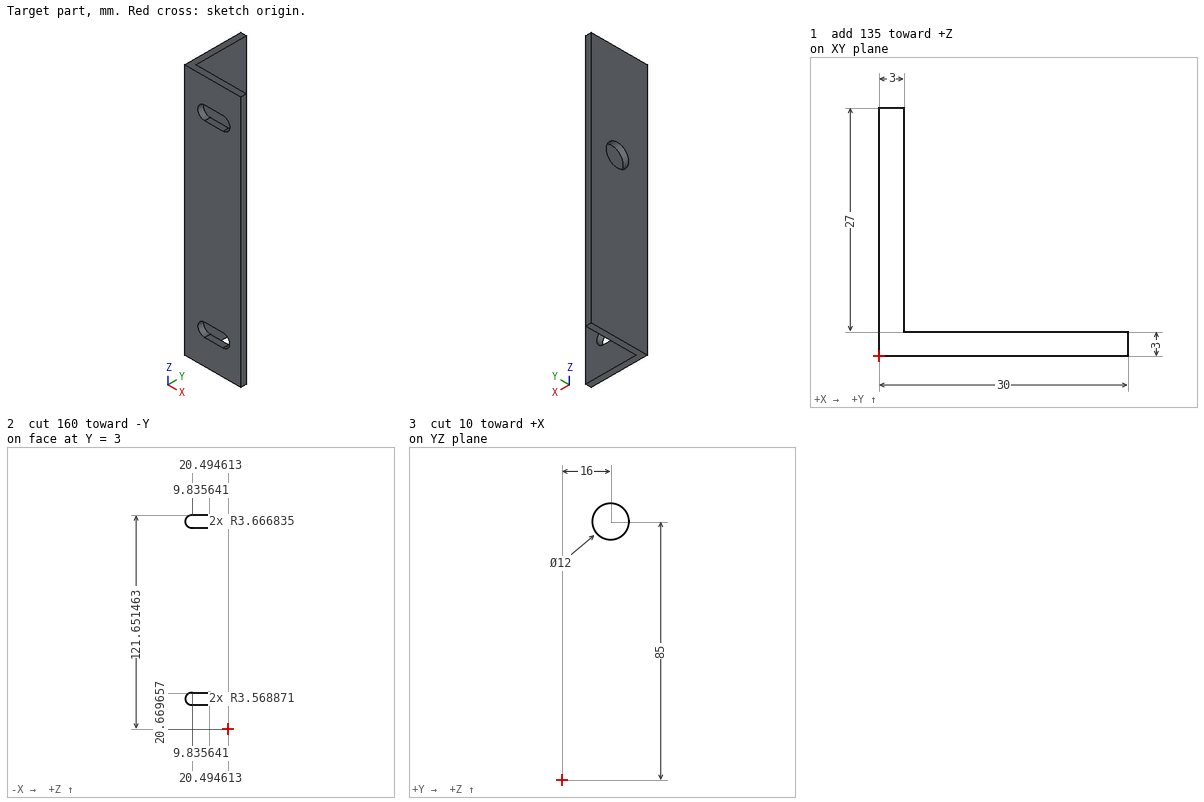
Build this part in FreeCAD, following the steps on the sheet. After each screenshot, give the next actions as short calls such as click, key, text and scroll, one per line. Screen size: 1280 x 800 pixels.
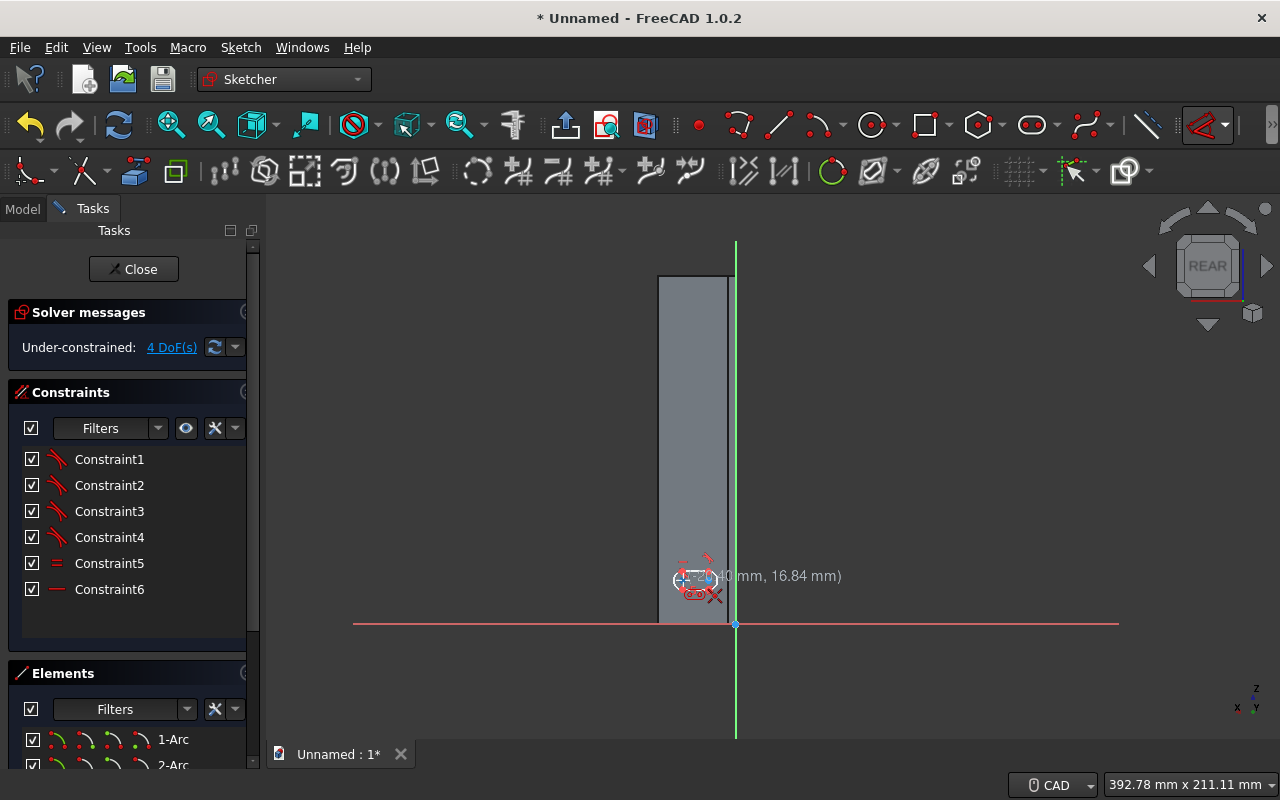
scroll(683, 320, up, 5)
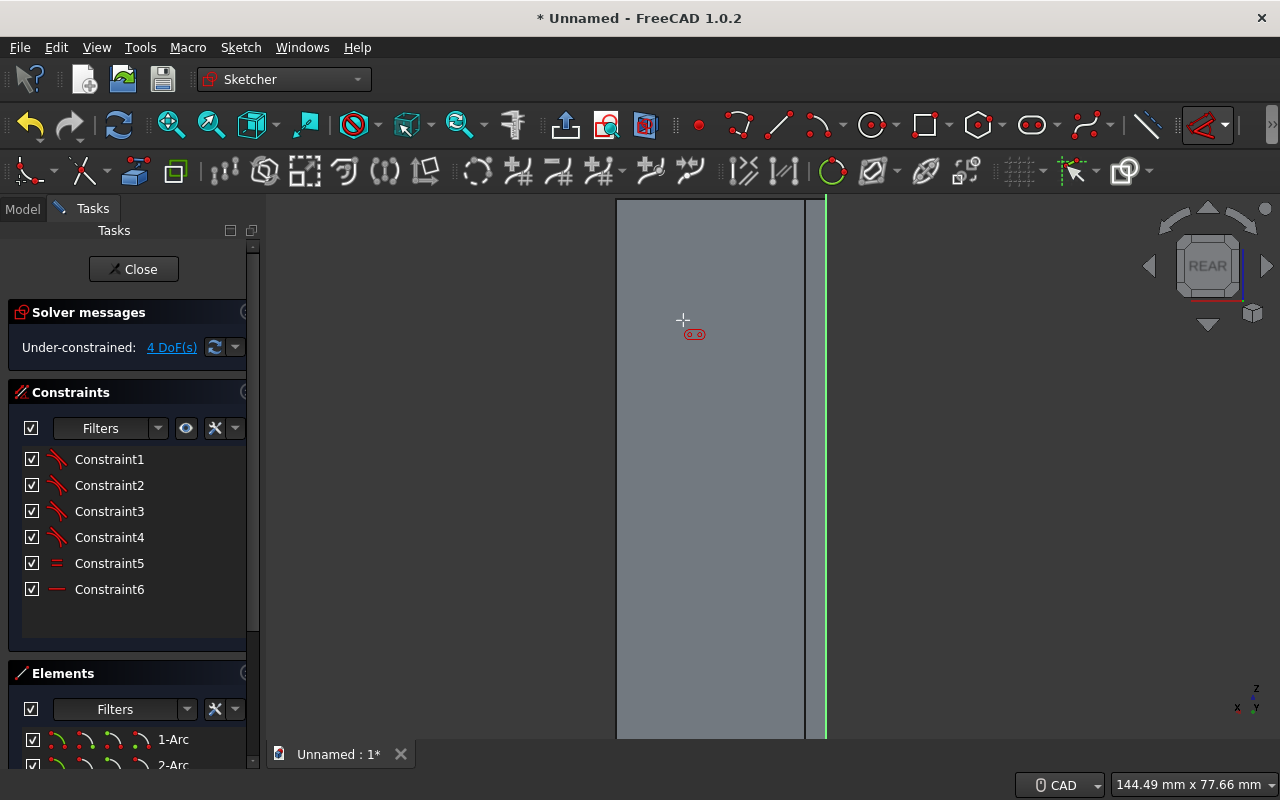
click(682, 319)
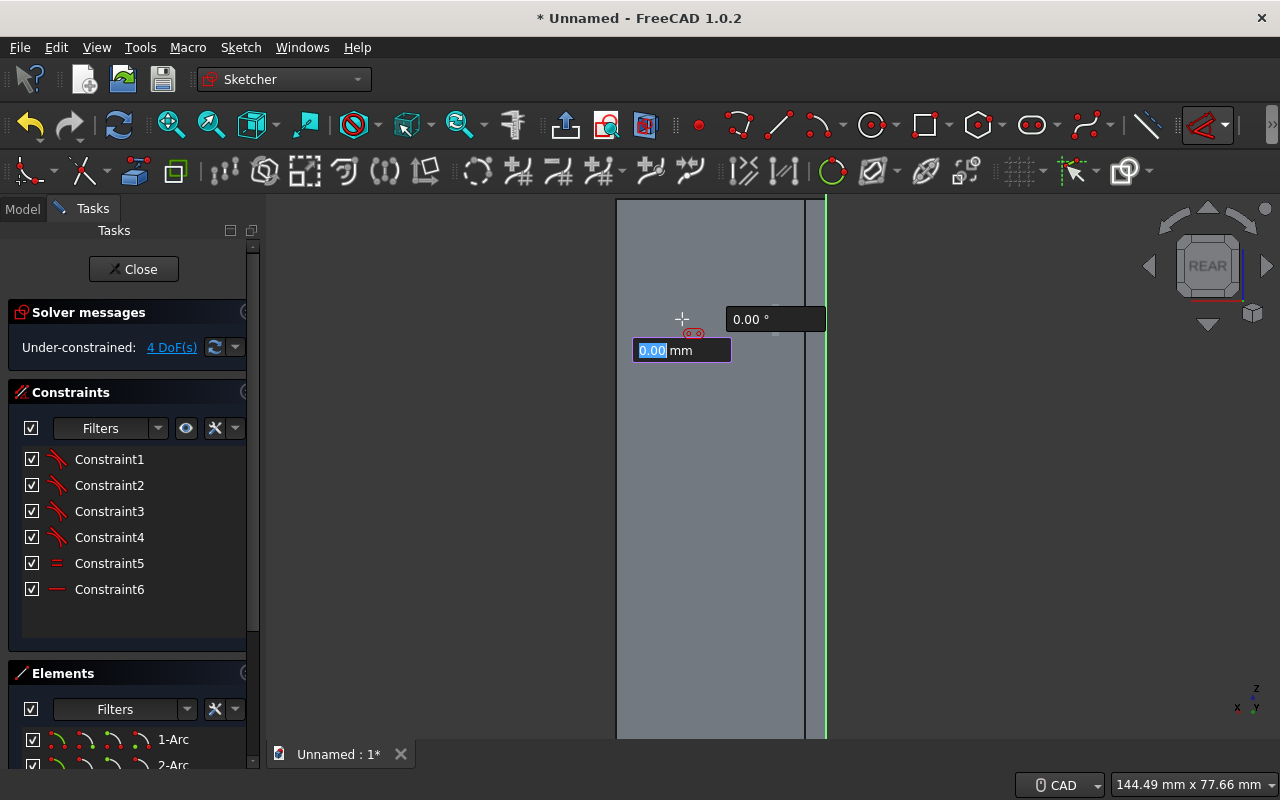
click(751, 319)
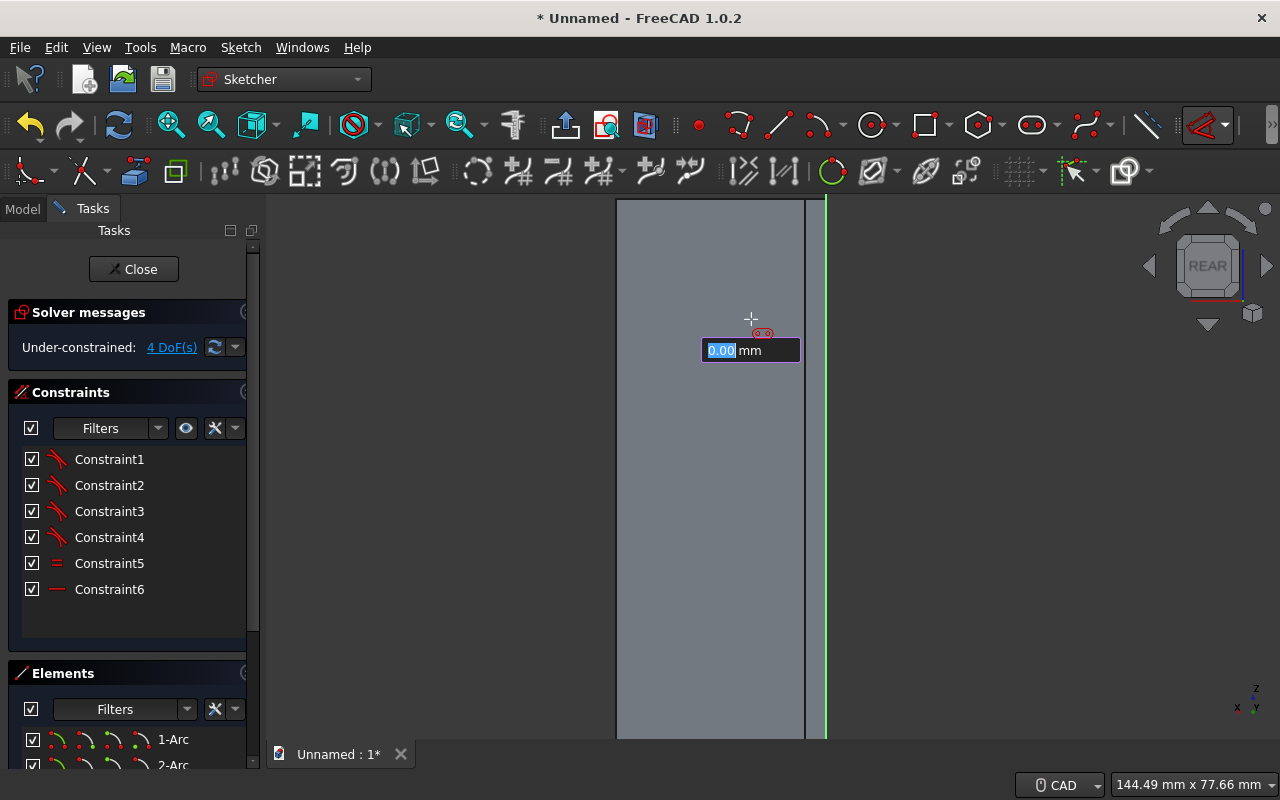
click(717, 344)
key(Escape)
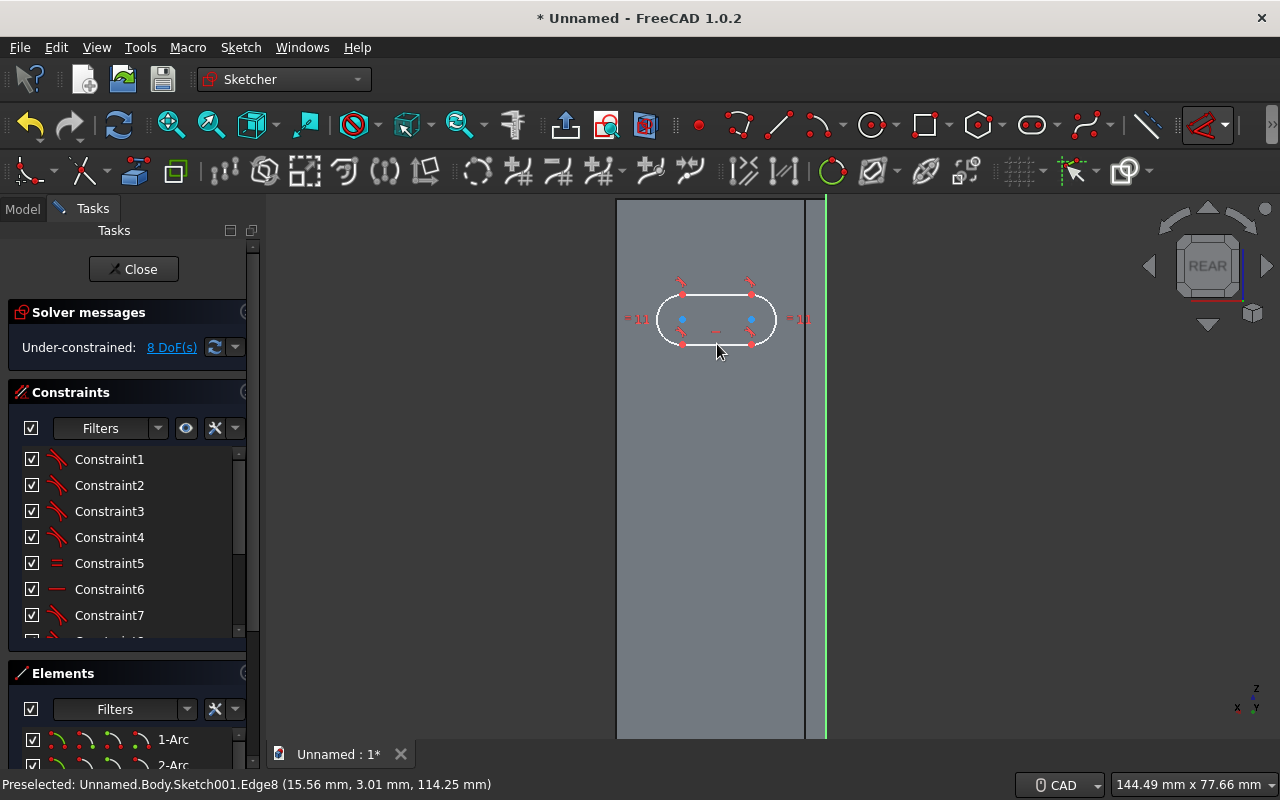
scroll(683, 319, down, 5)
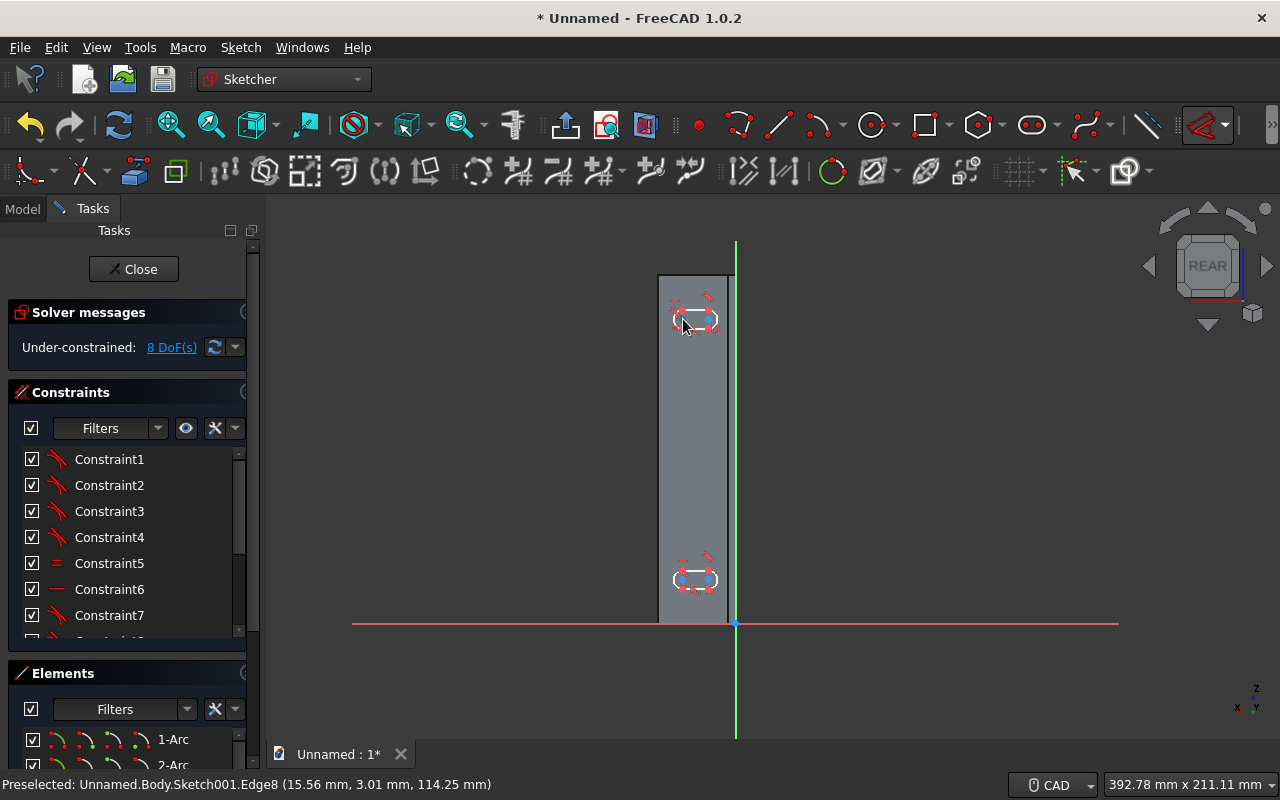
scroll(675, 574, up, 8)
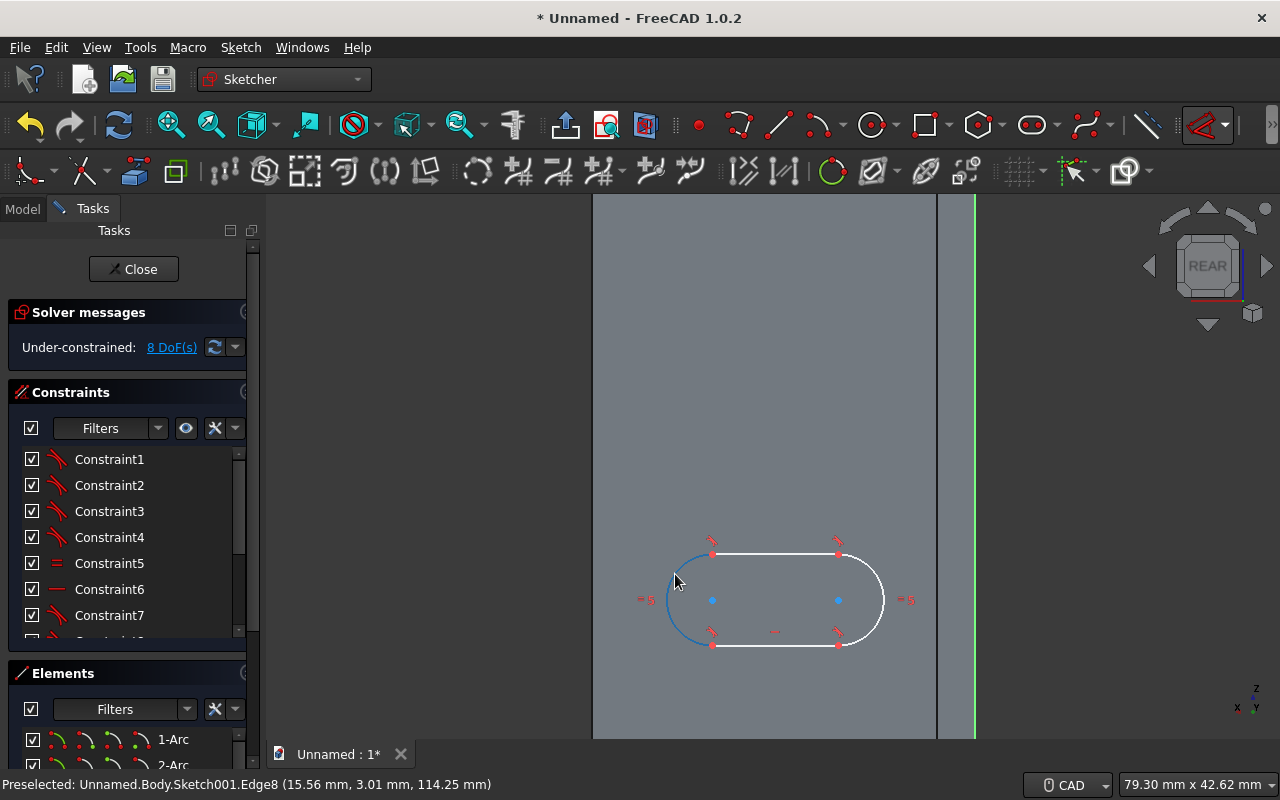
click(676, 573)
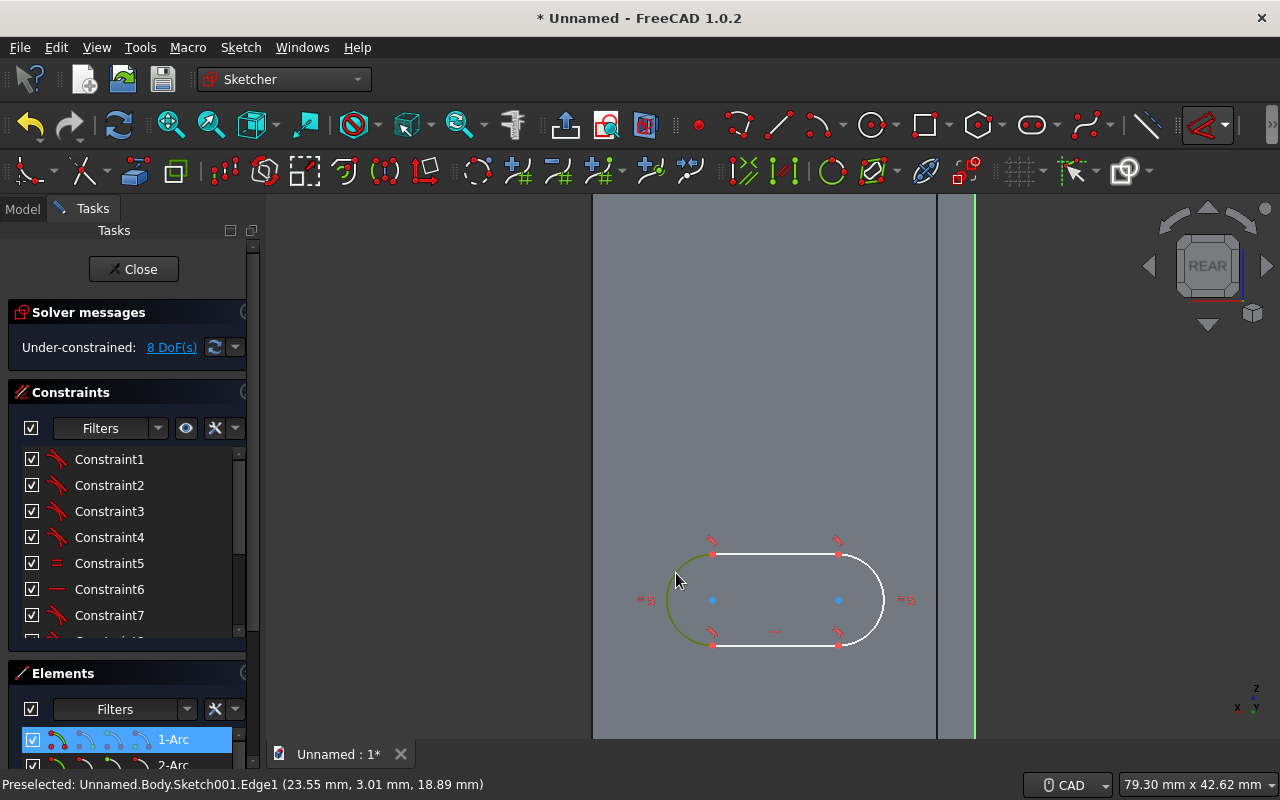
key(k)
key(r)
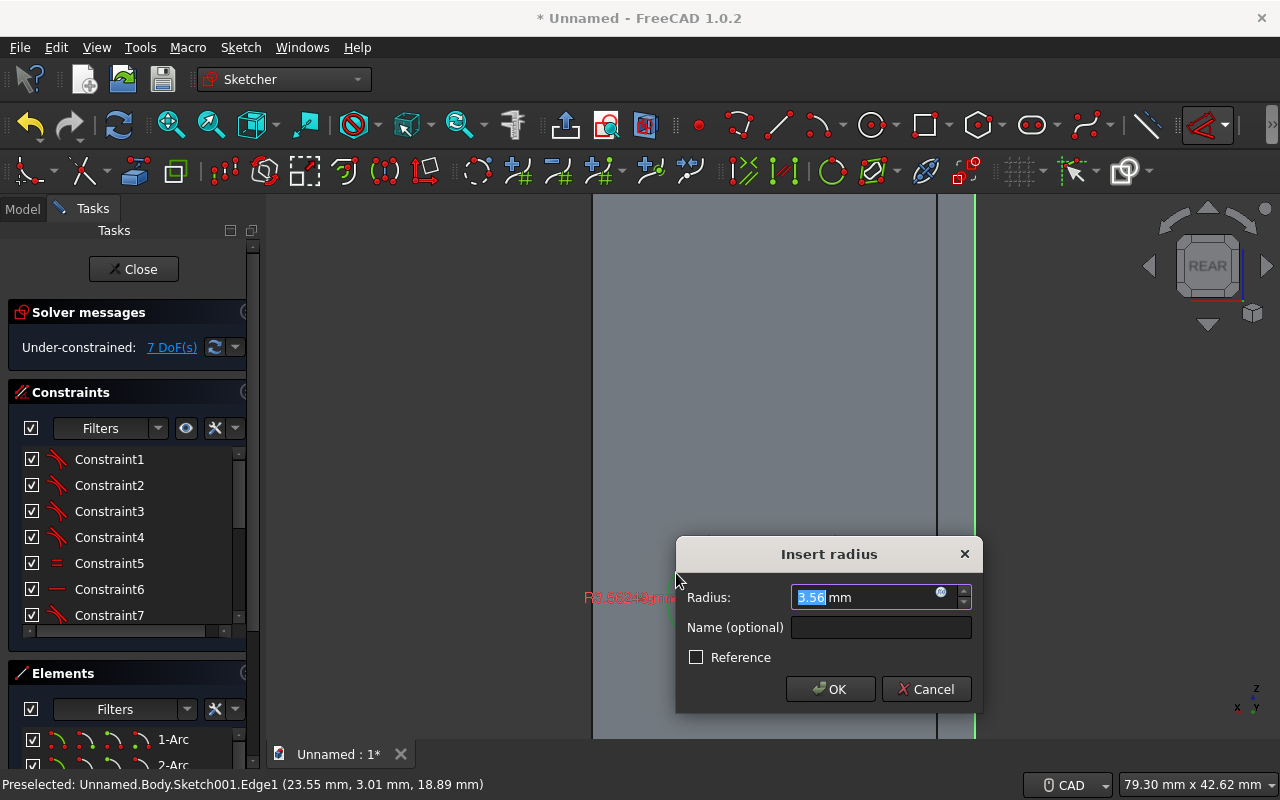
text(3.568871)
key(Return)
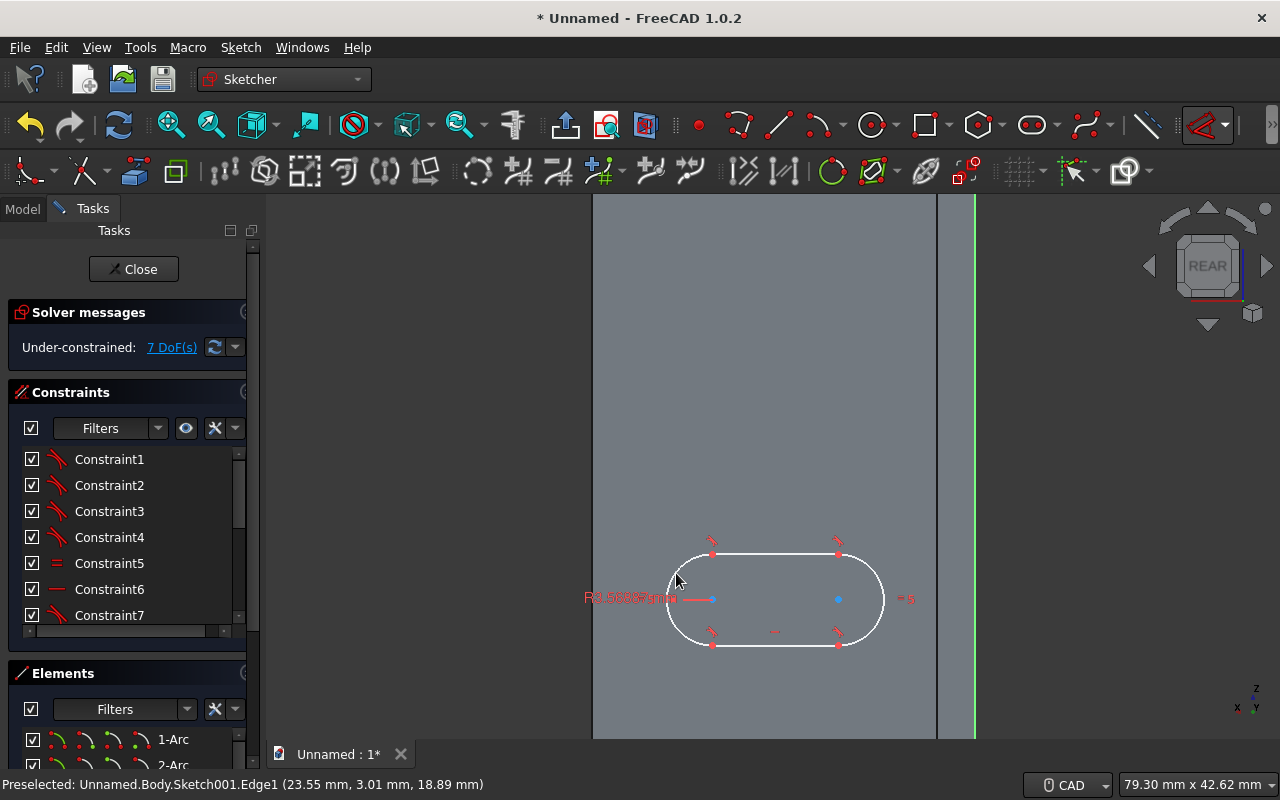
scroll(675, 575, down, 8)